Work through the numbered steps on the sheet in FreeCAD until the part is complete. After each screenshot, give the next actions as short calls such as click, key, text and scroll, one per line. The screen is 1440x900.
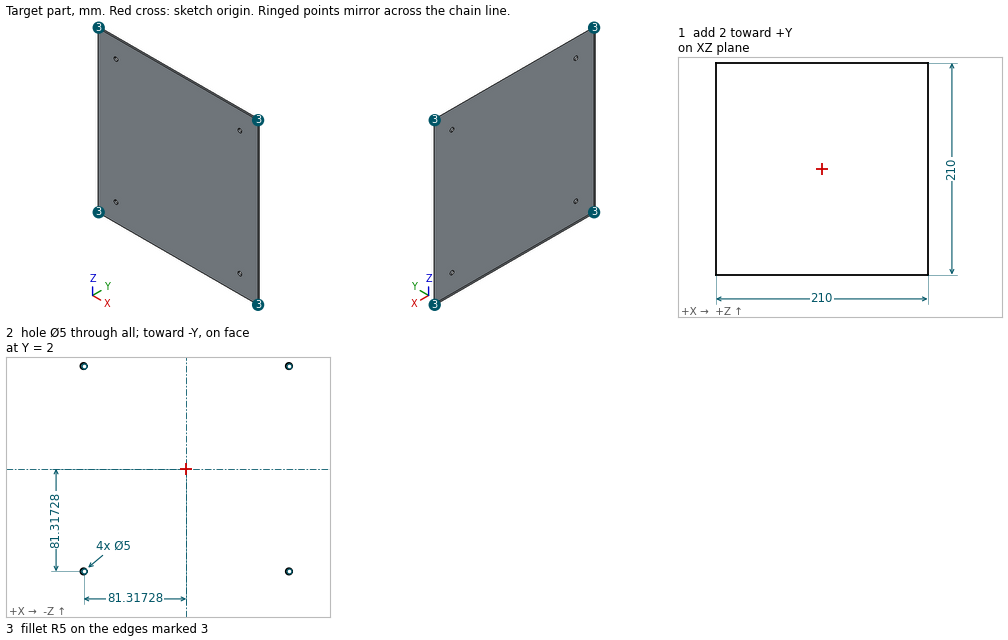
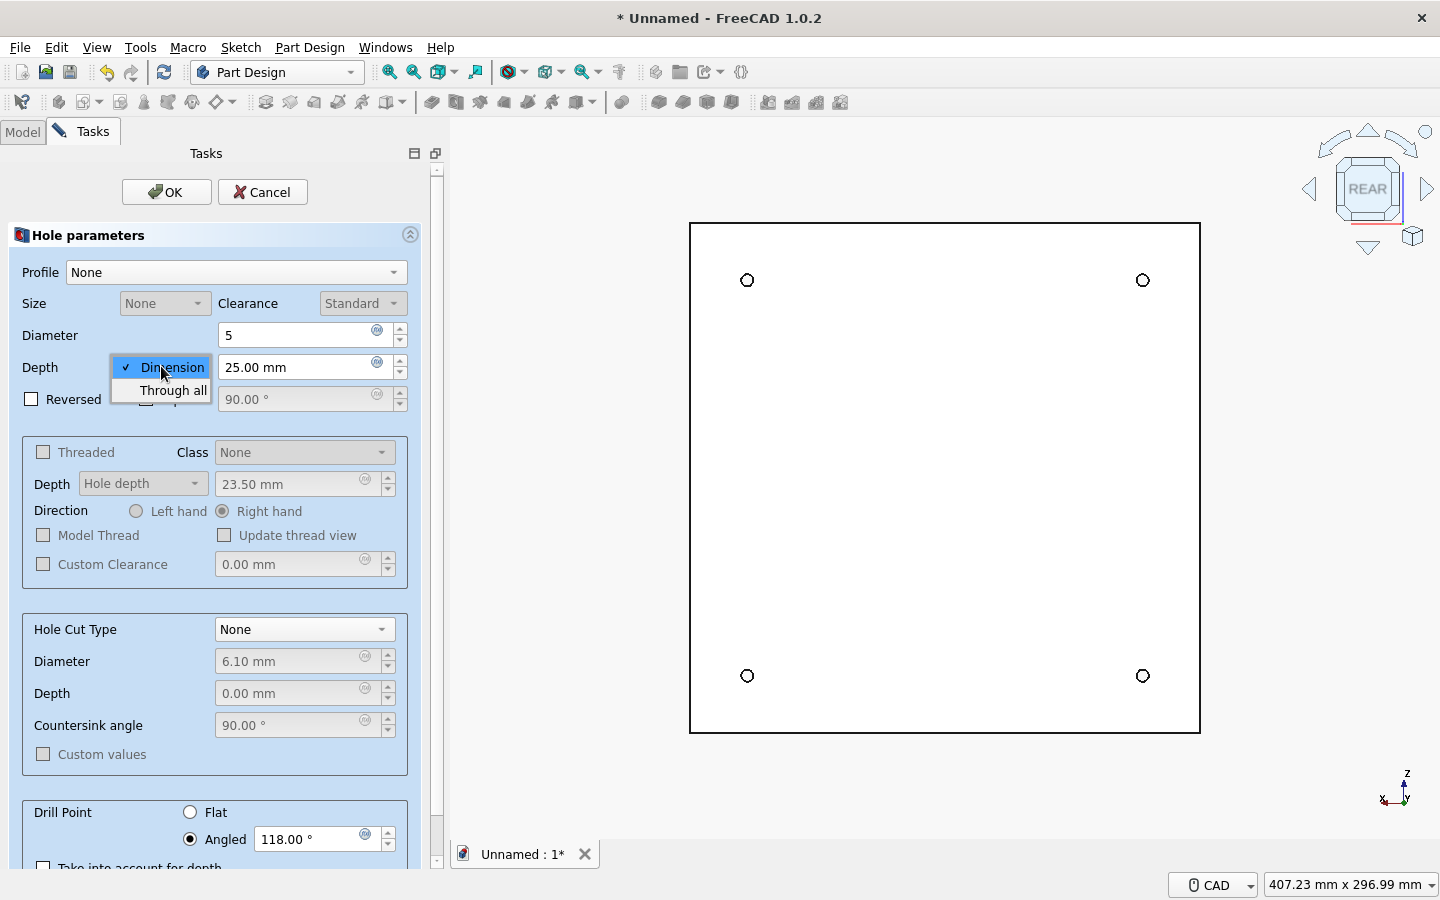
click(160, 390)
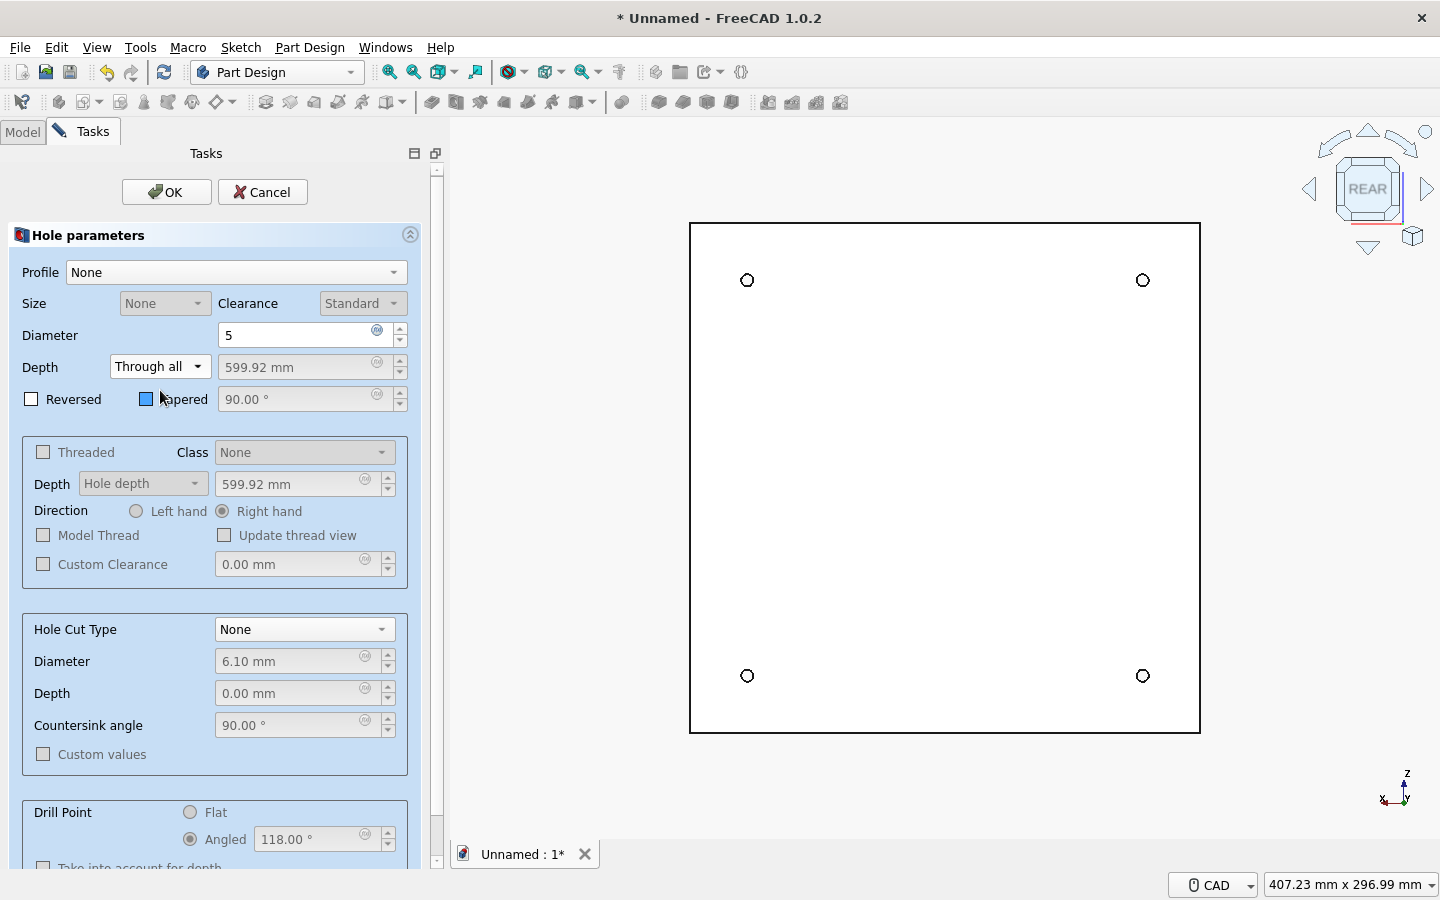
click(167, 192)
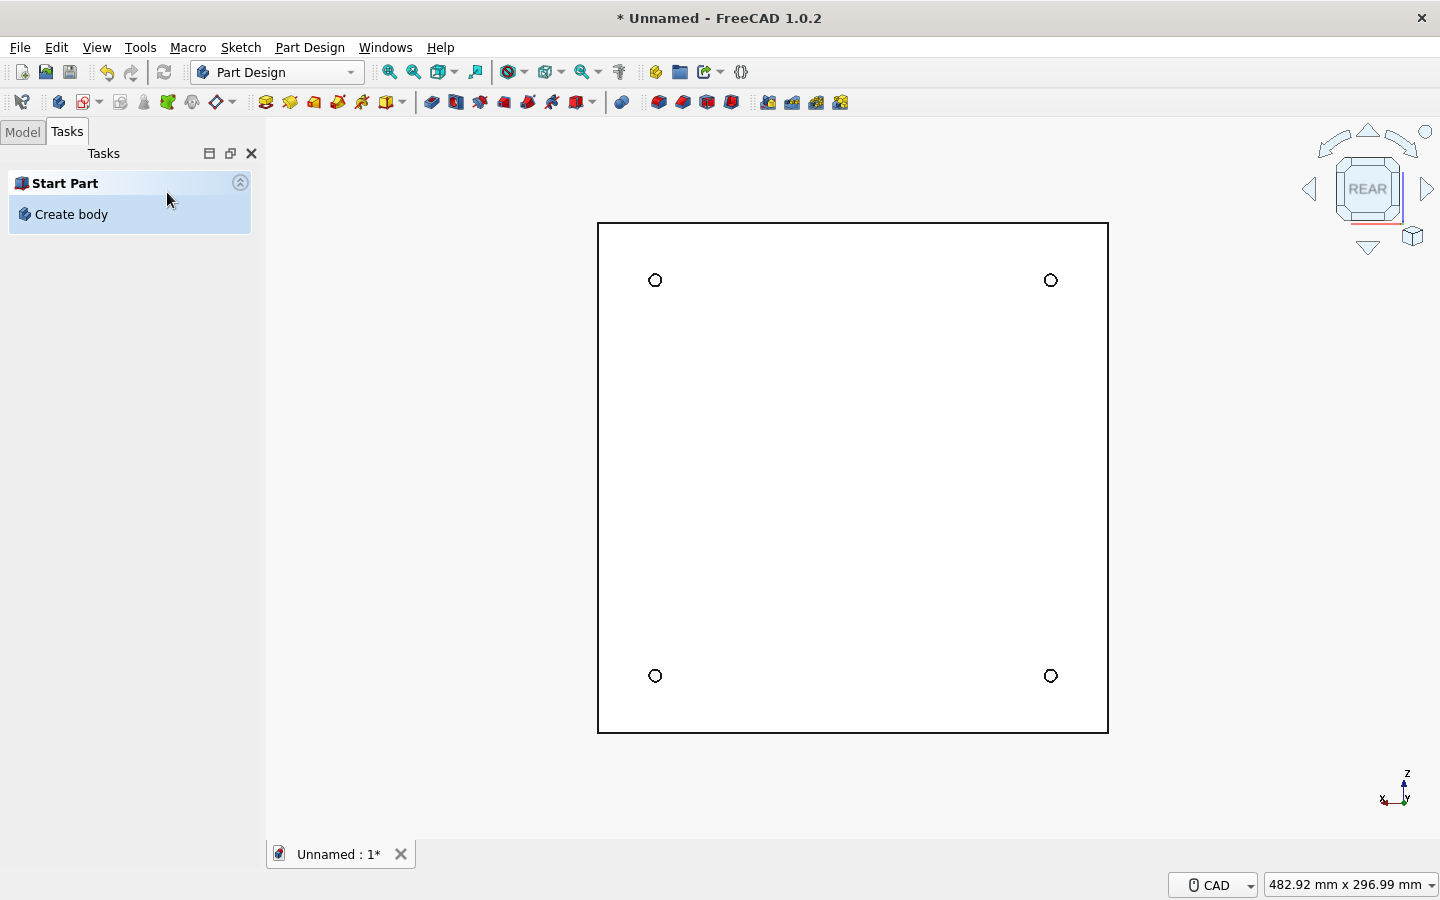
scroll(598, 222, up, 11)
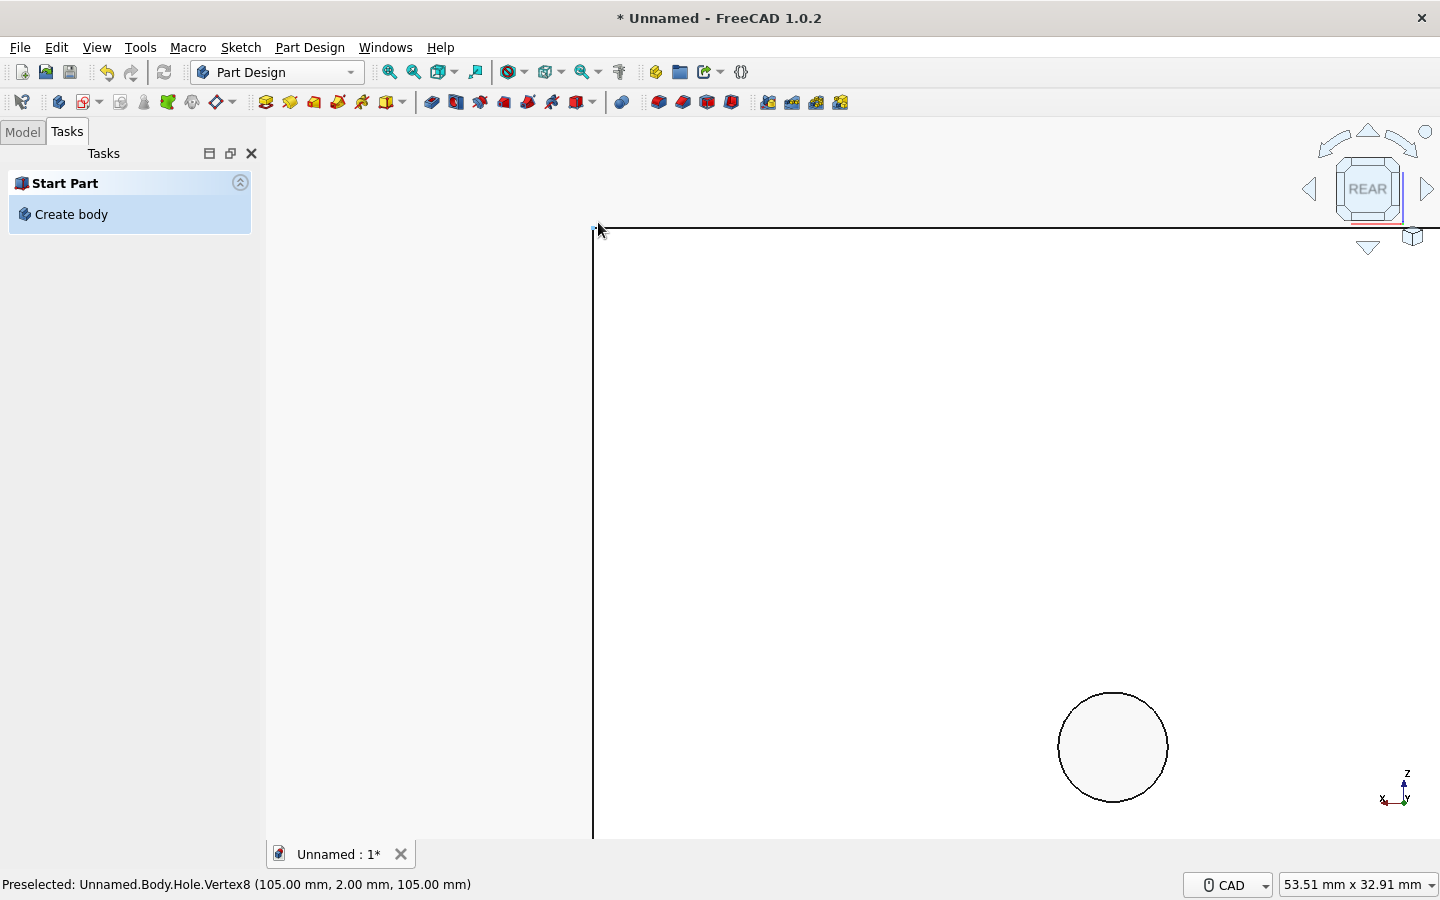
click(390, 72)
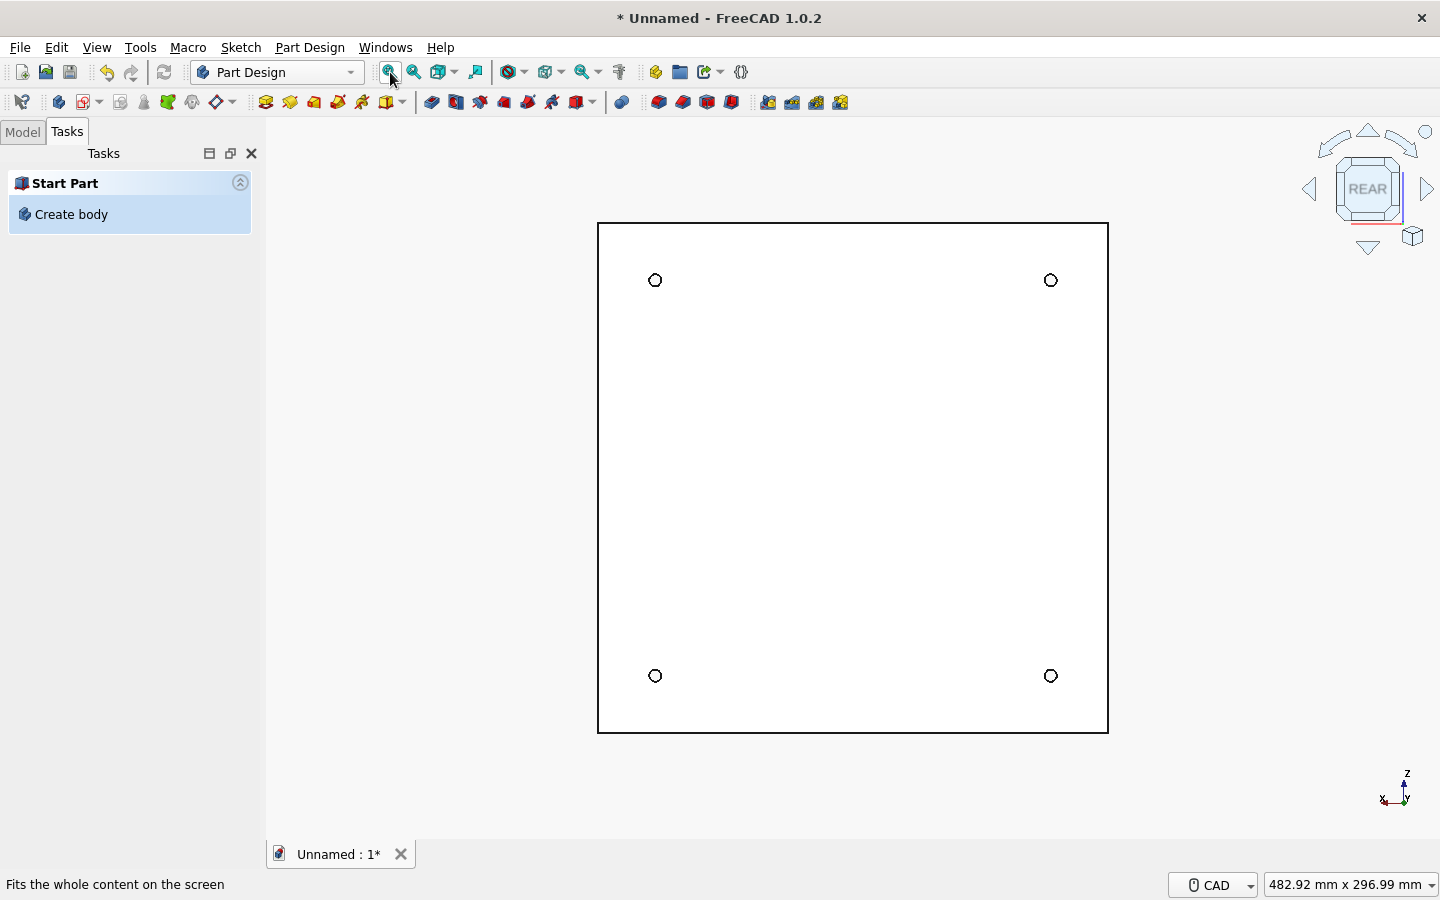
key(0)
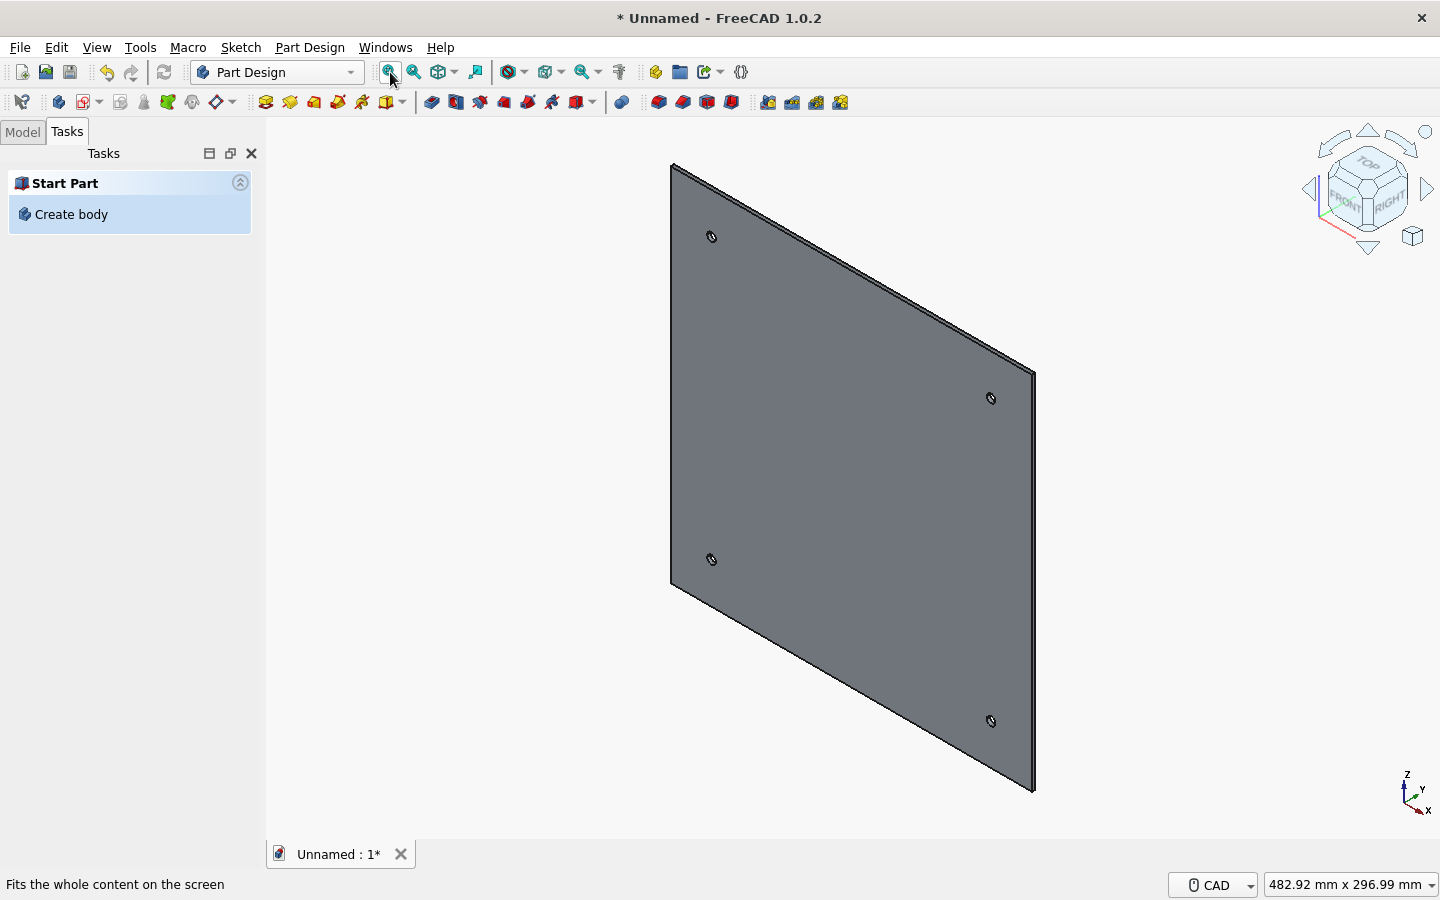
scroll(1033, 373, up, 11)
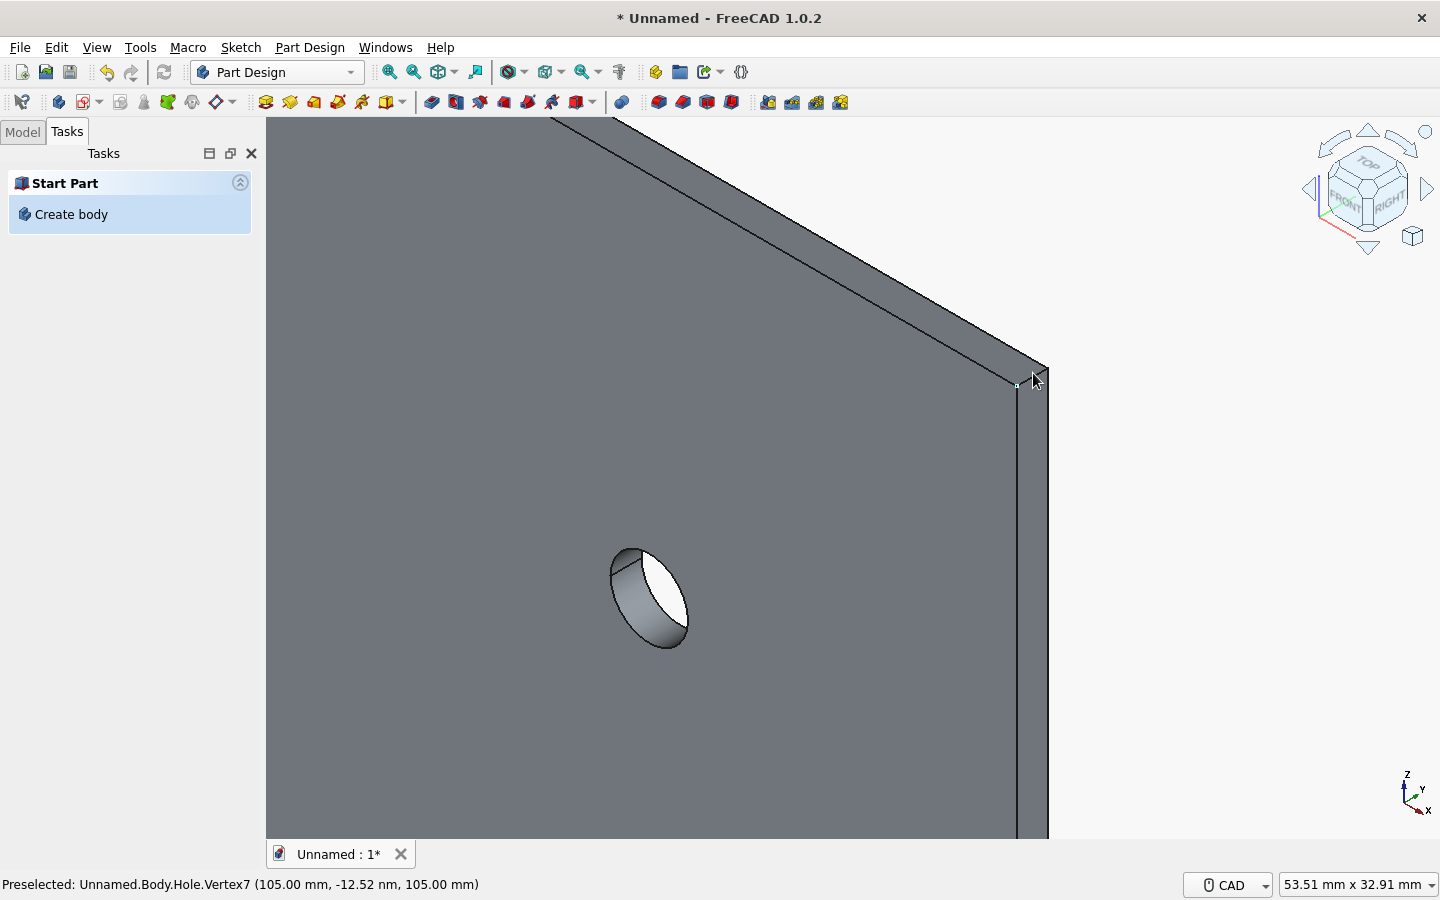
click(1032, 376)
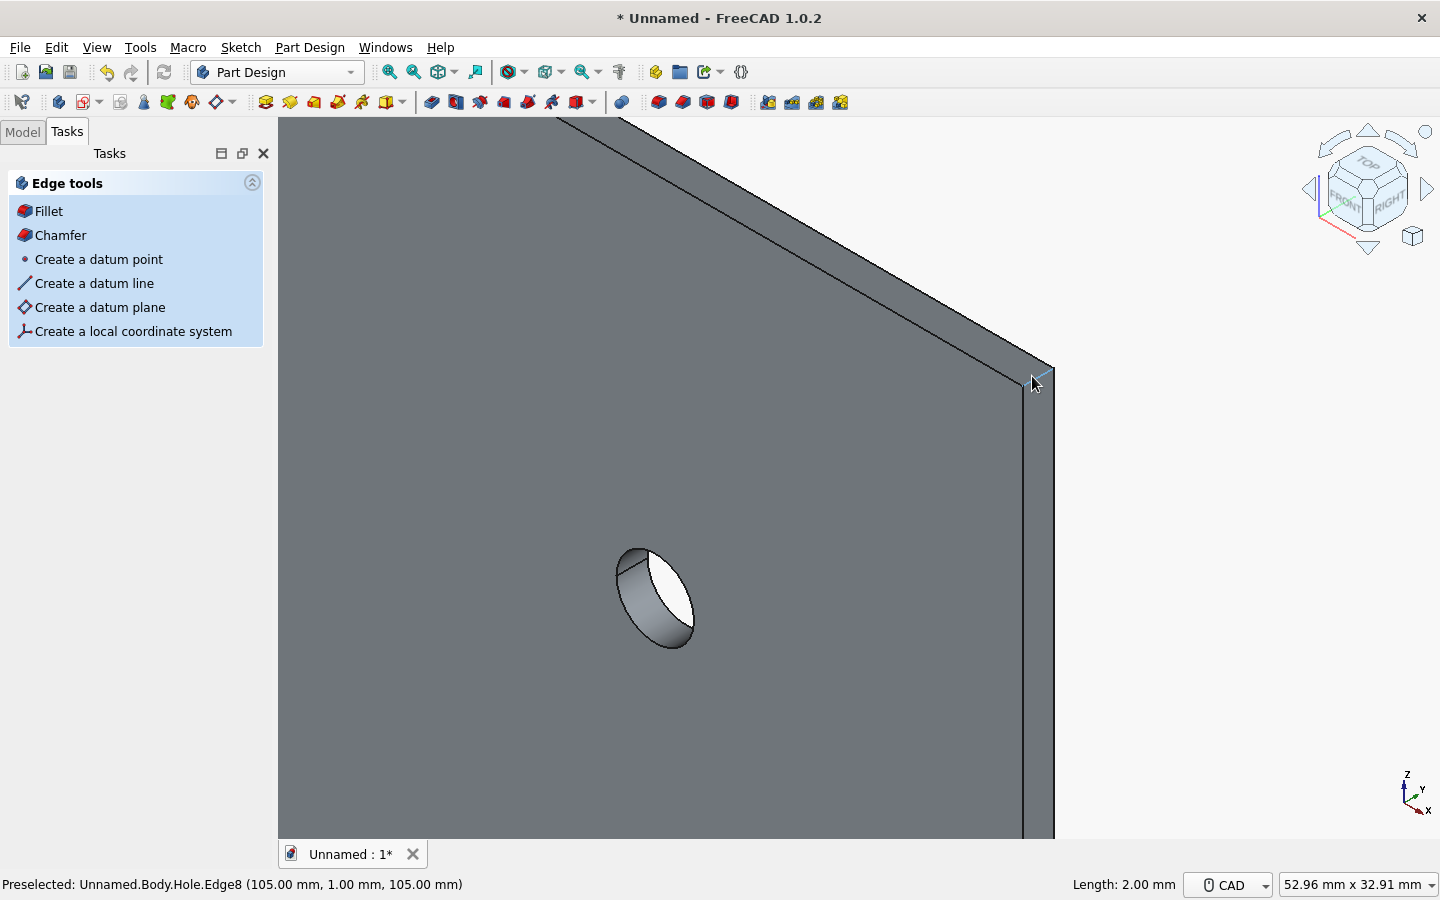
click(390, 72)